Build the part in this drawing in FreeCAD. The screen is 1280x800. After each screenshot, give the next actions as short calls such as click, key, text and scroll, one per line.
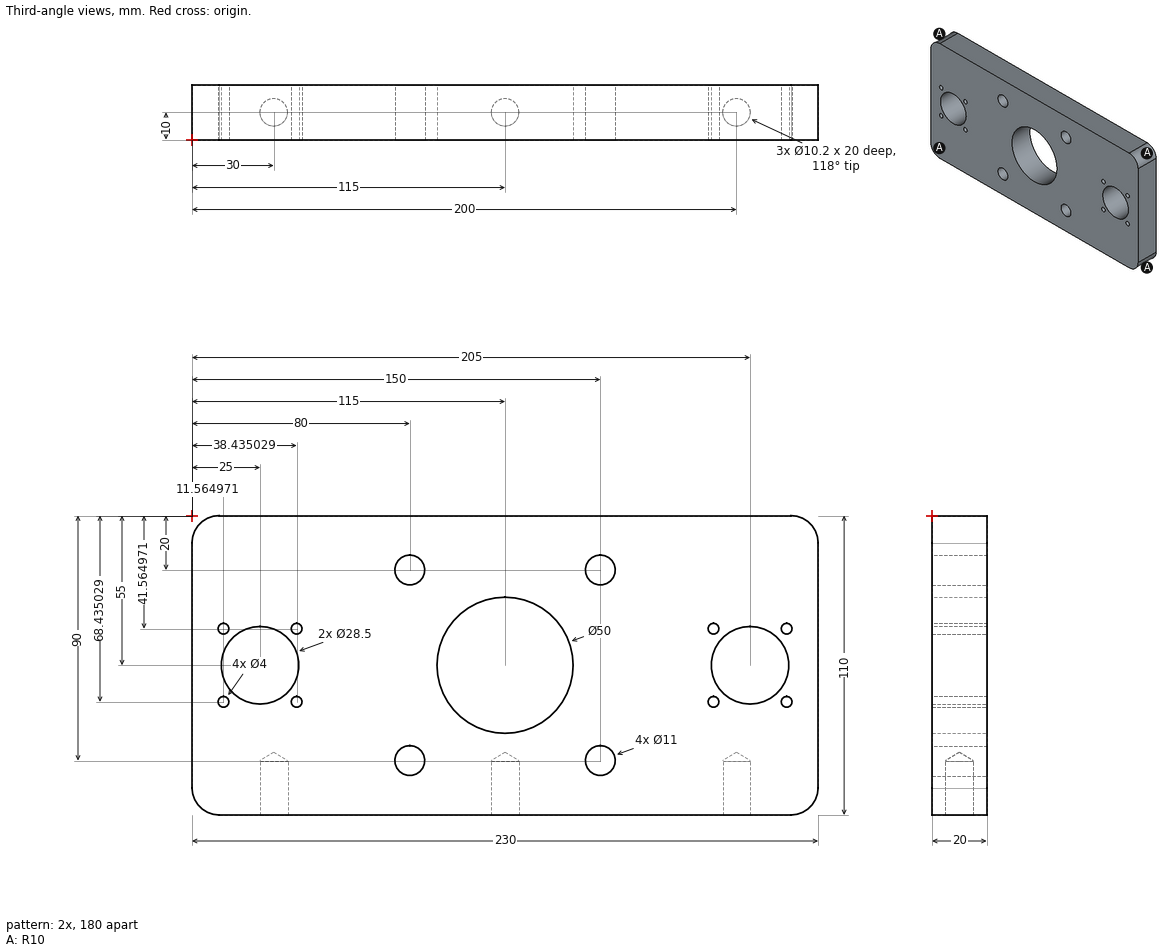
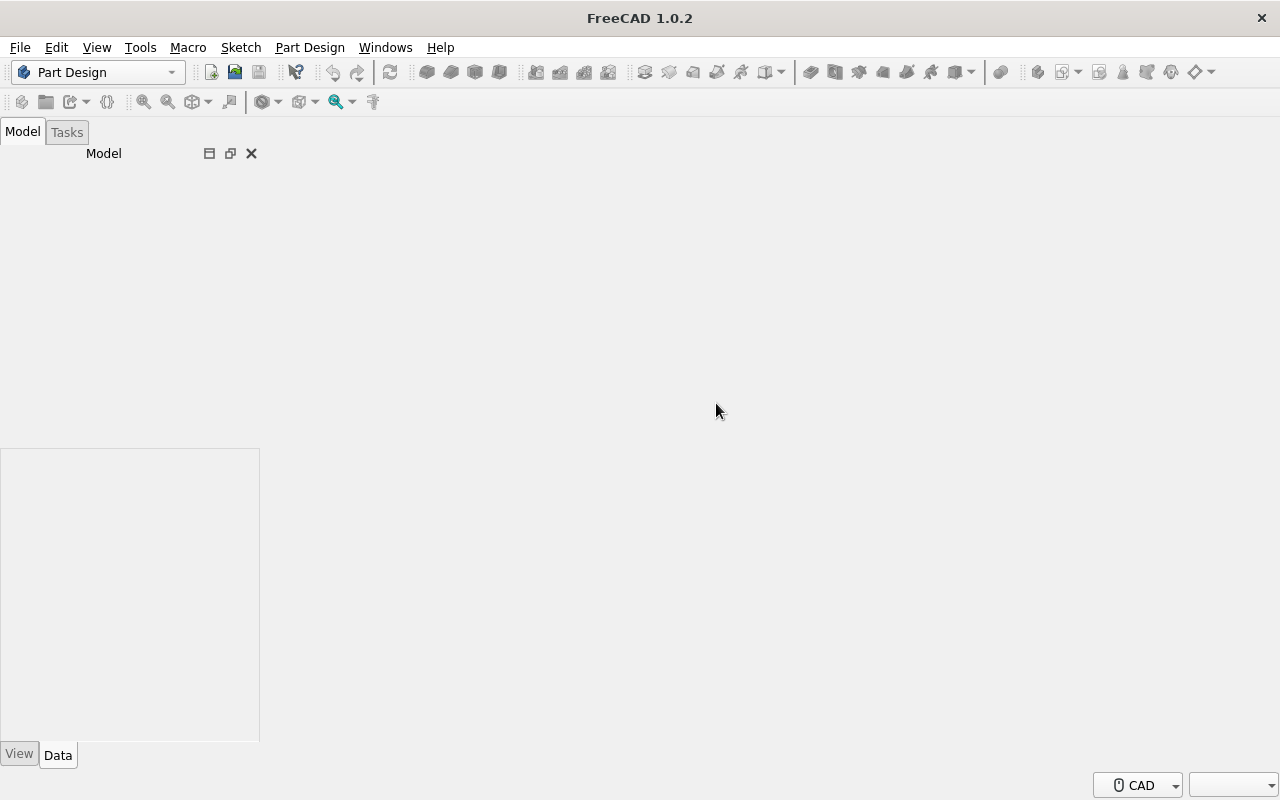
key(ctrl+n)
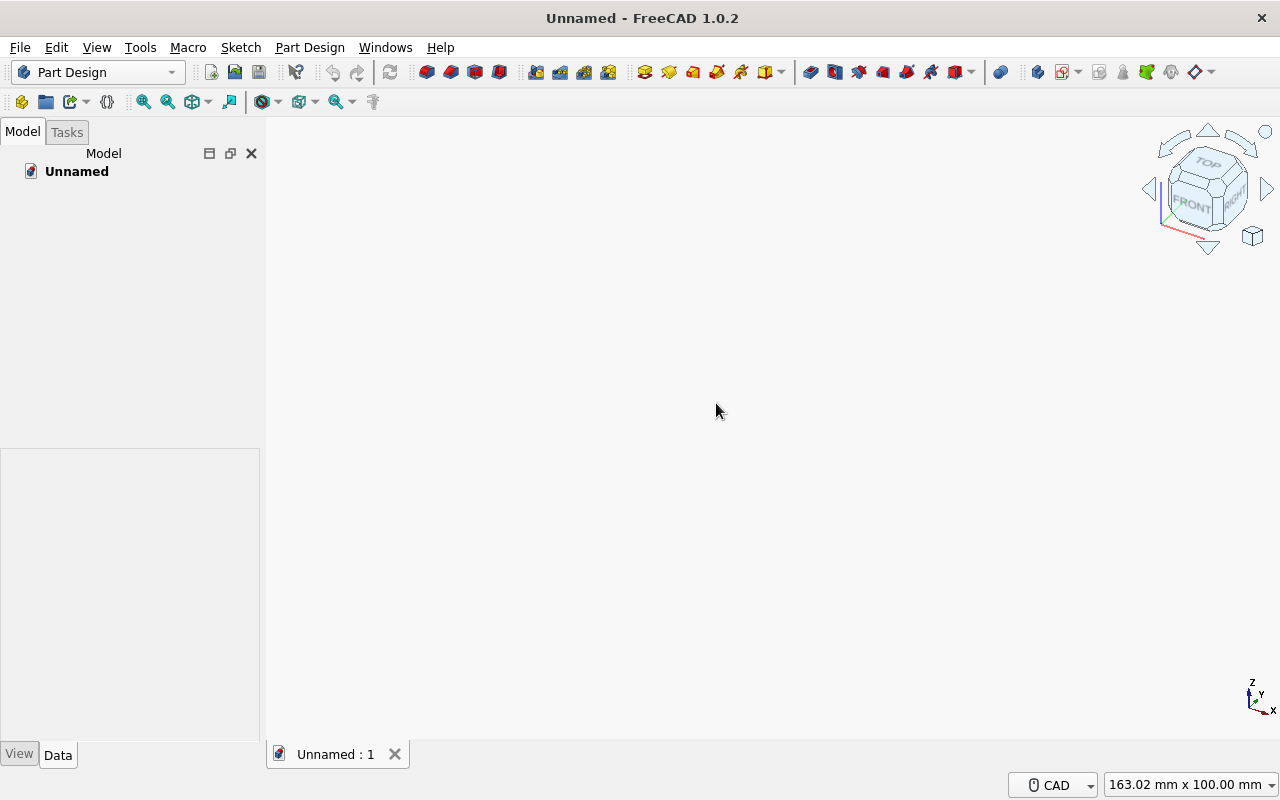
click(1062, 72)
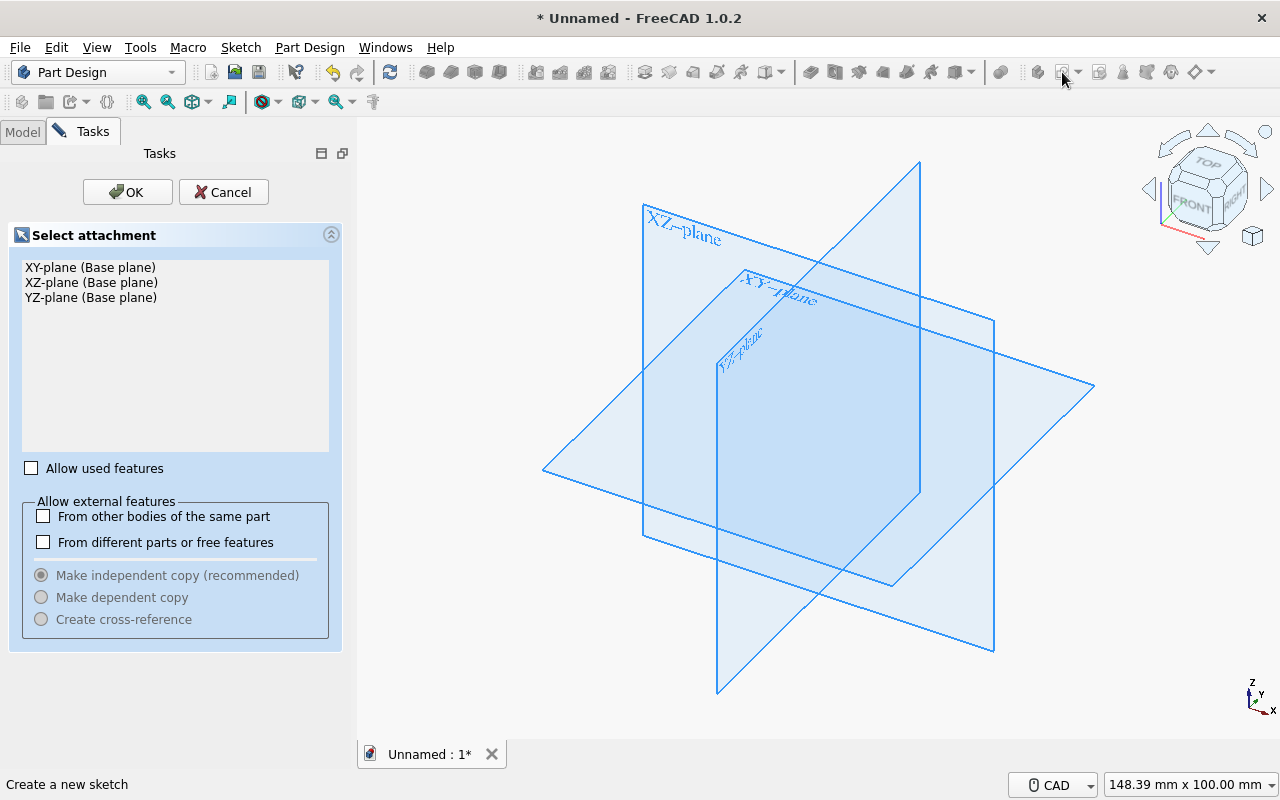
click(82, 282)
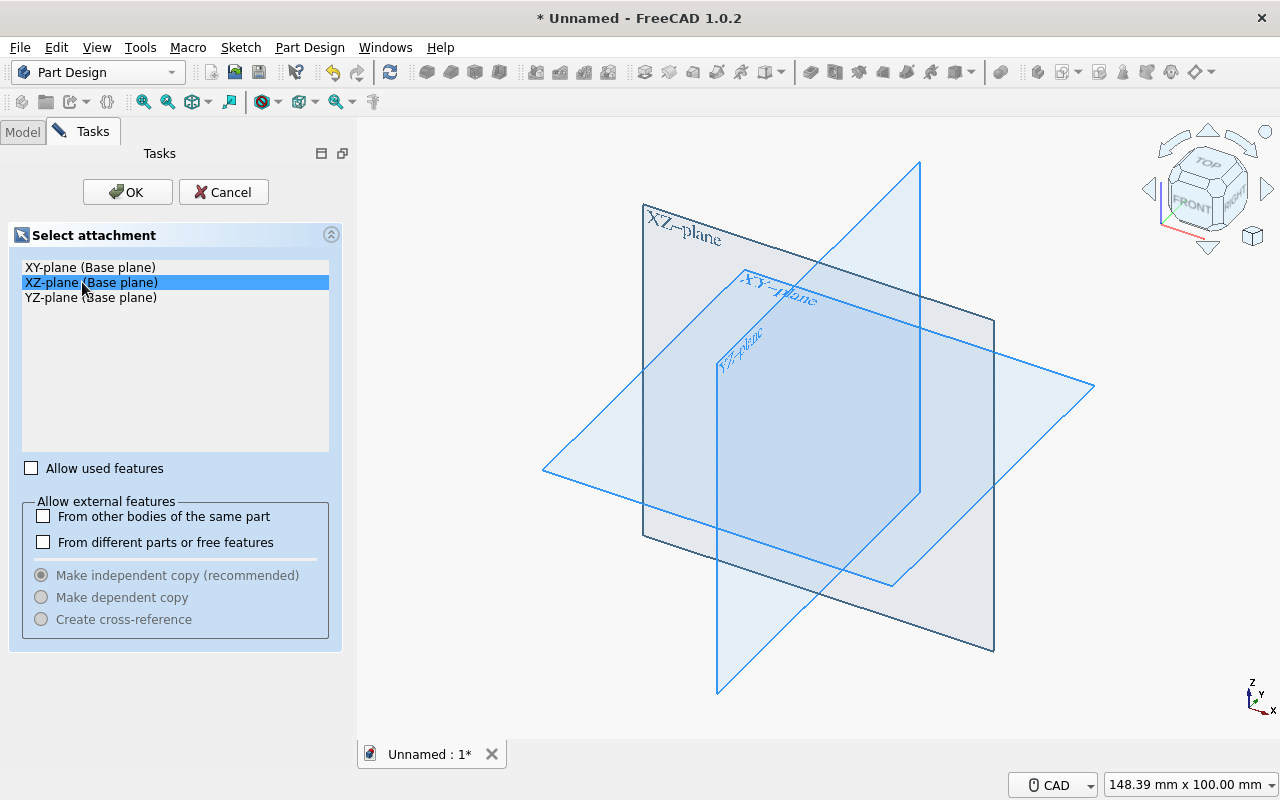
click(128, 192)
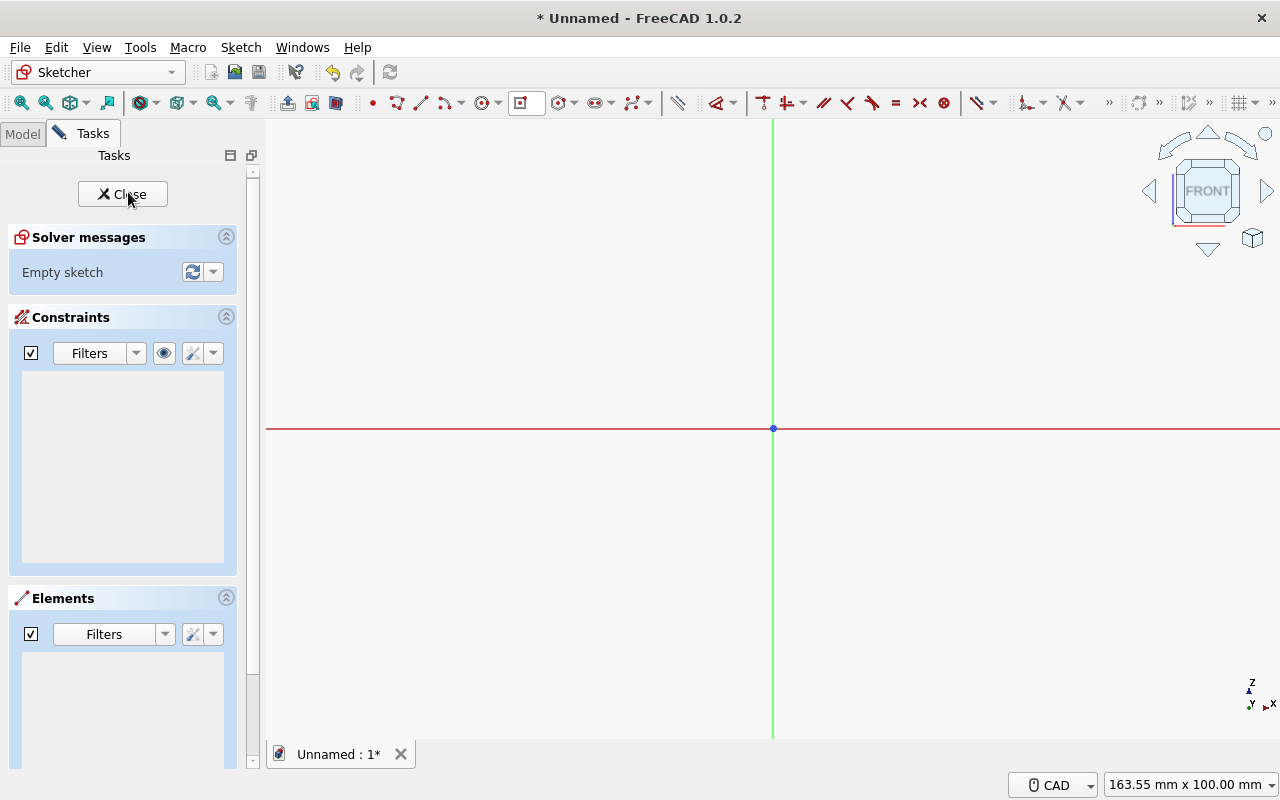
scroll(294, 231, down, 5)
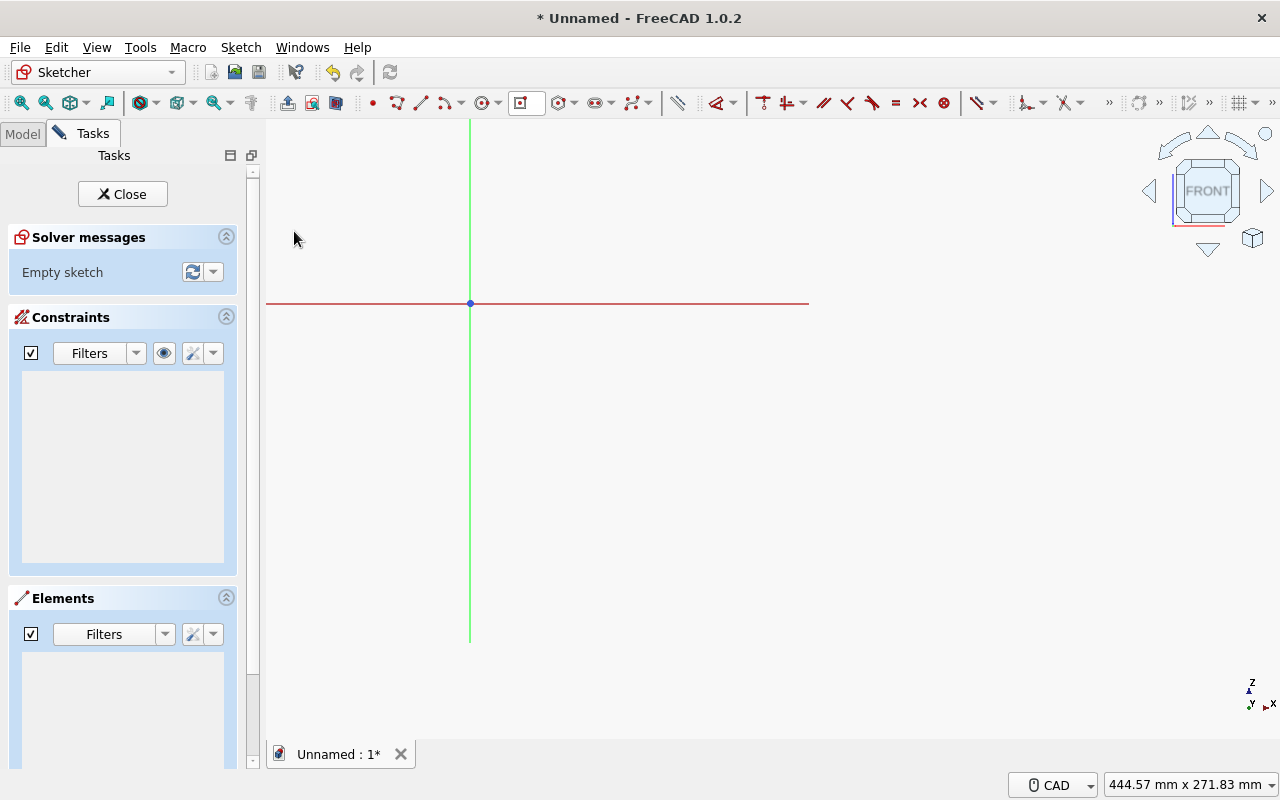
key(g)
key(r)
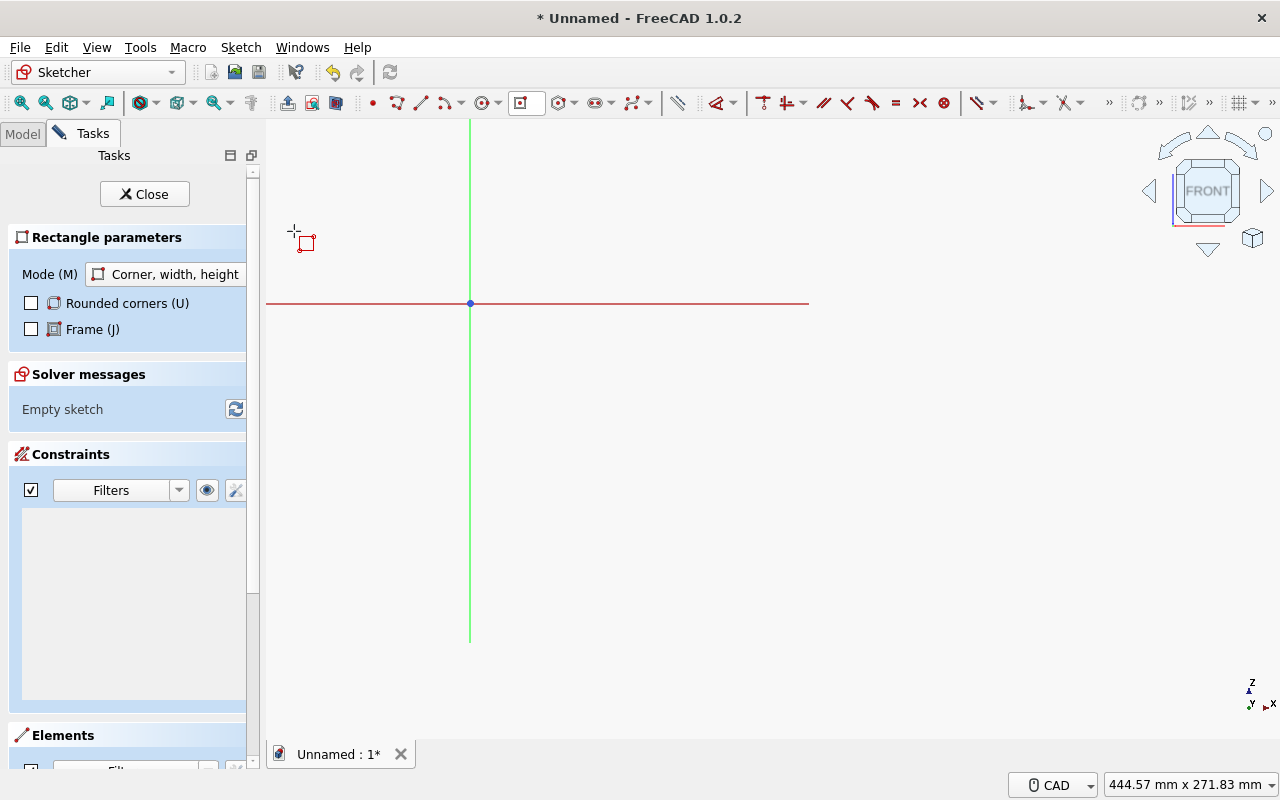
click(470, 304)
move(995, 555)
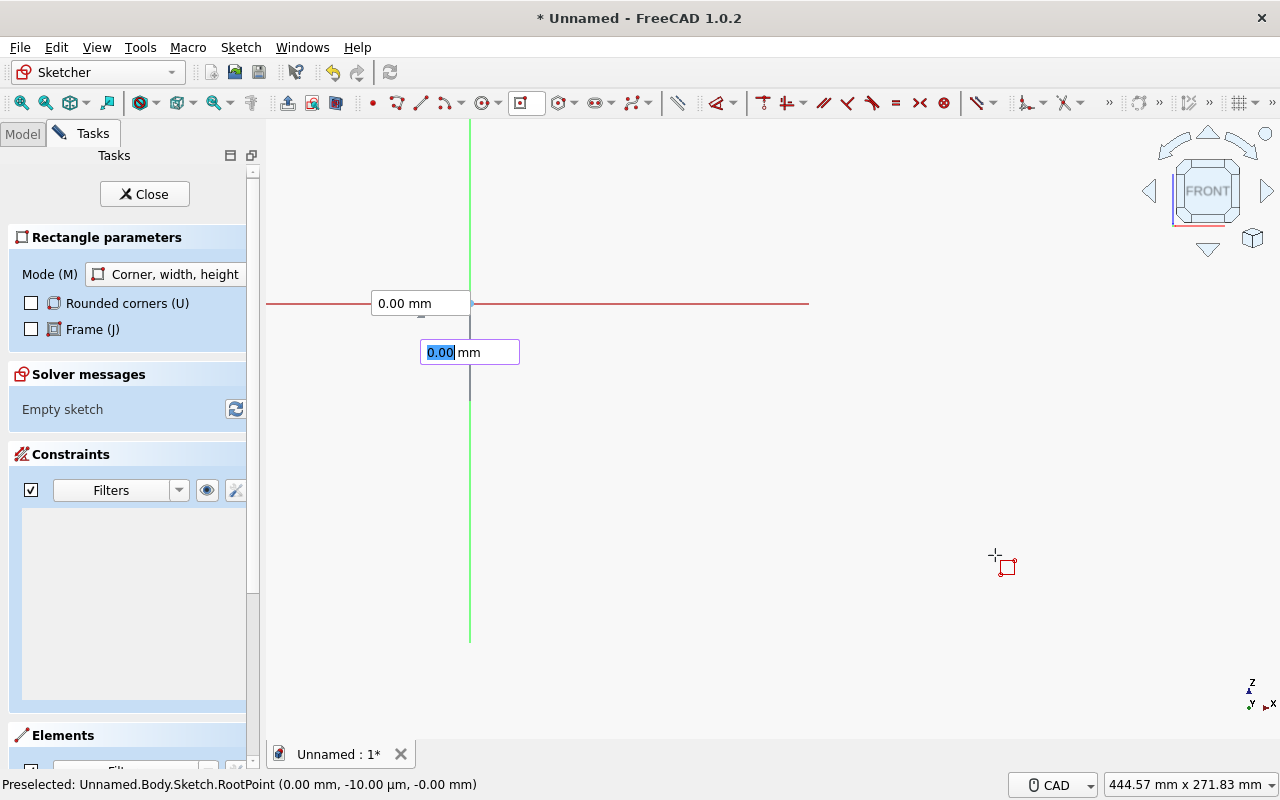
text(230)
key(Tab)
text(110)
key(Return)
key(Escape)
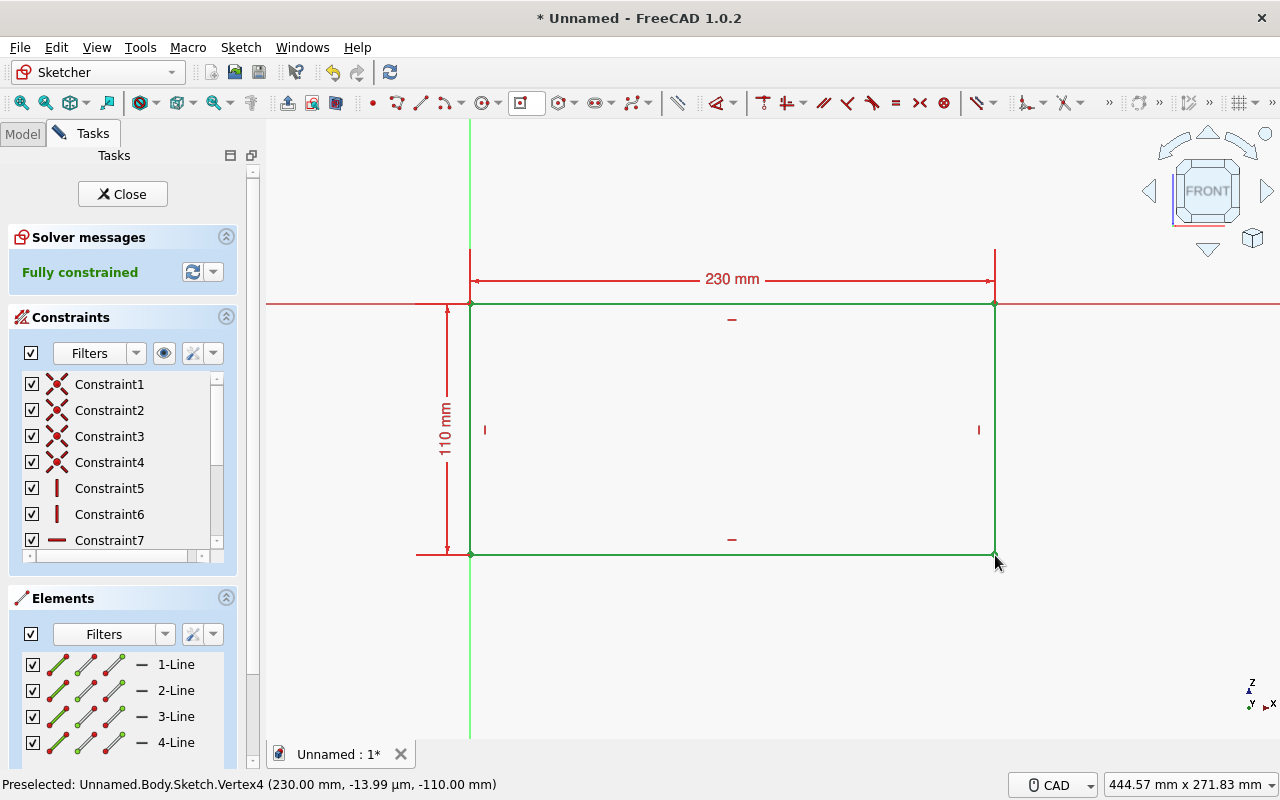
click(123, 194)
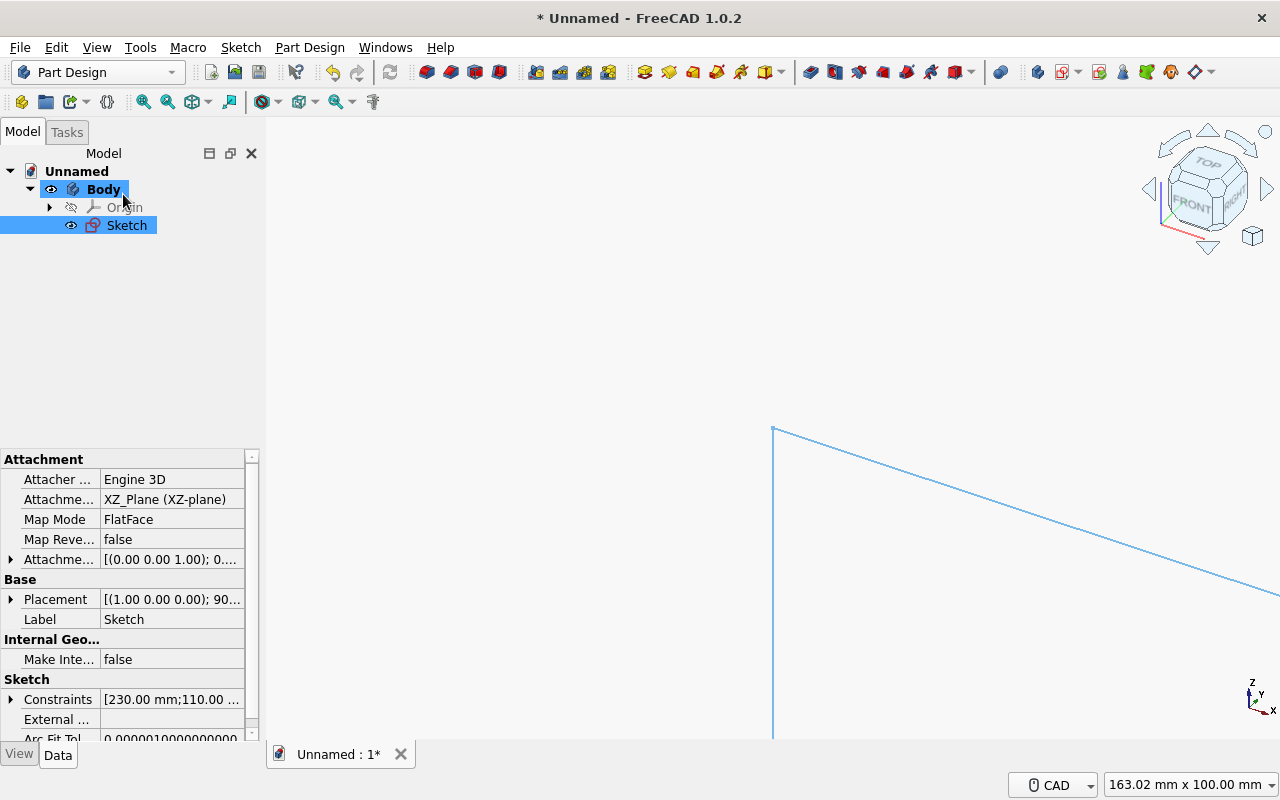
click(646, 72)